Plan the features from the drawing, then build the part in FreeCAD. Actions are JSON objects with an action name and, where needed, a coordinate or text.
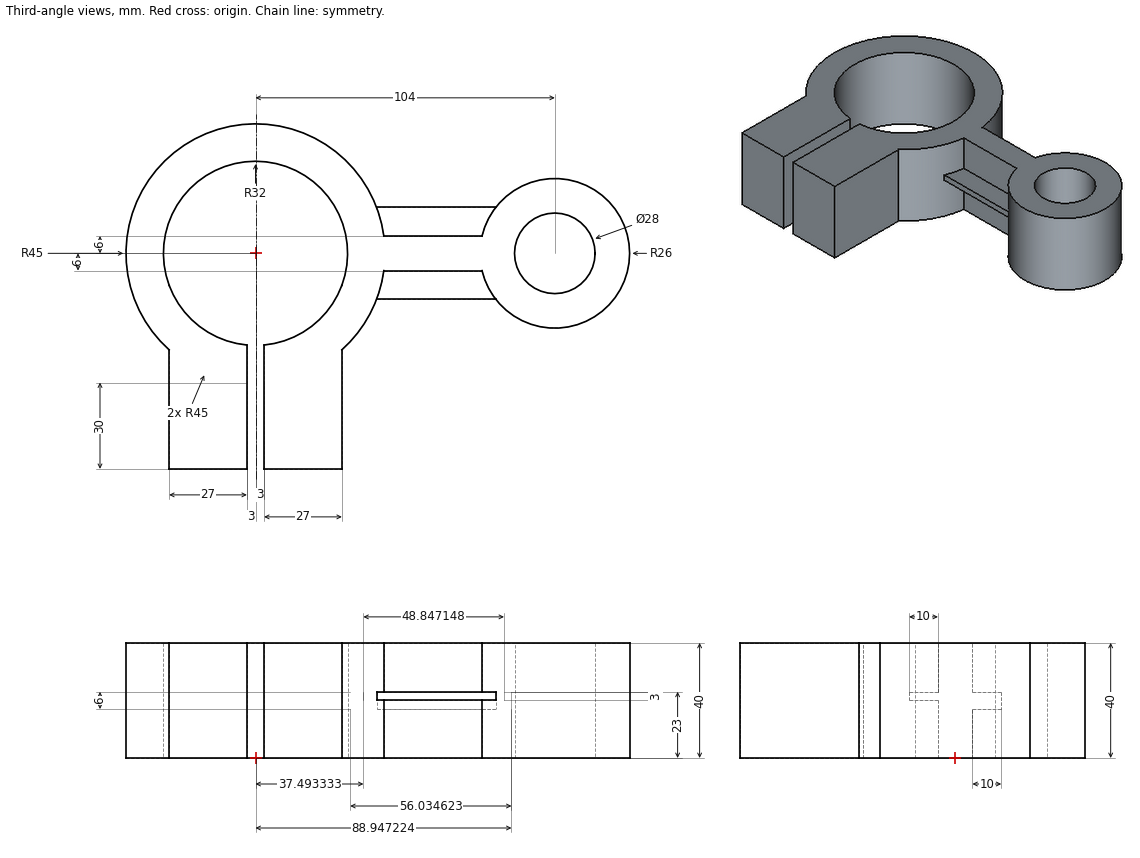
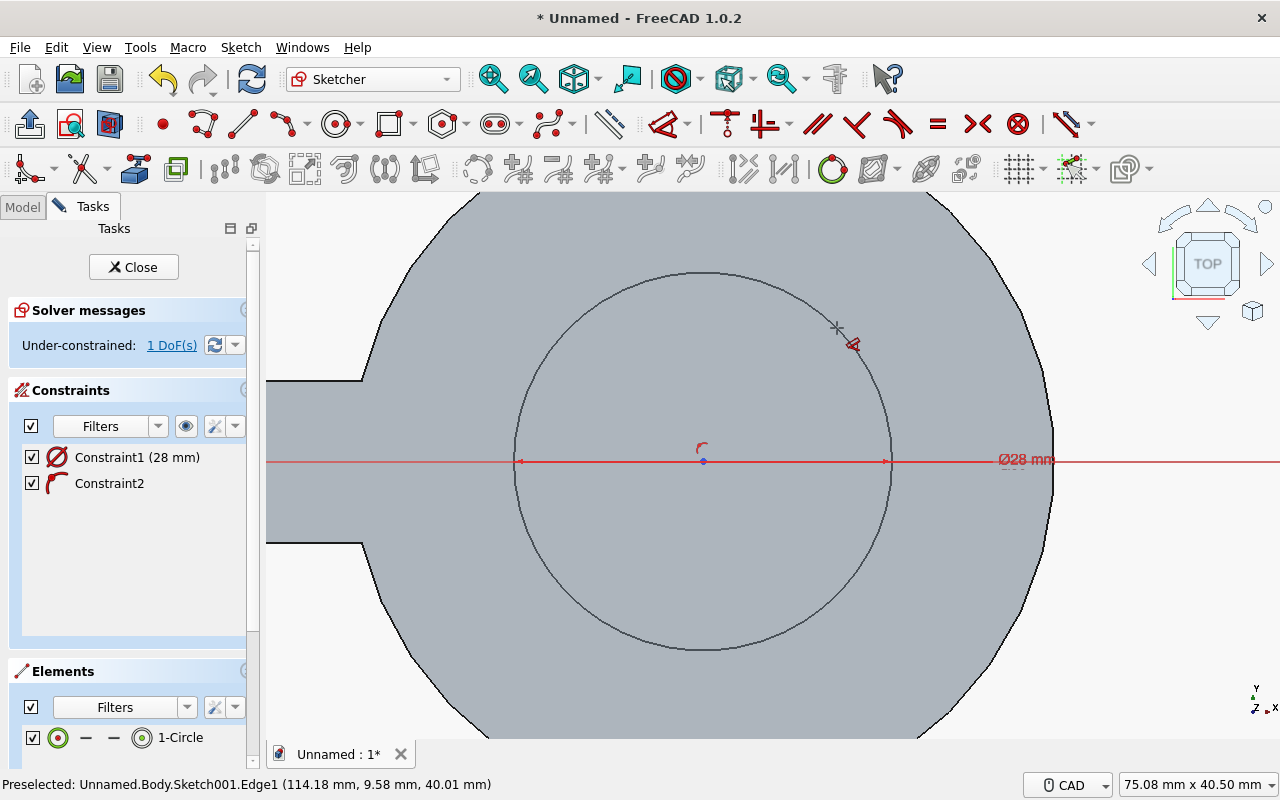
{"action": "left_click", "coordinate": [703, 462]}
{"action": "left_click", "coordinate": [498, 496]}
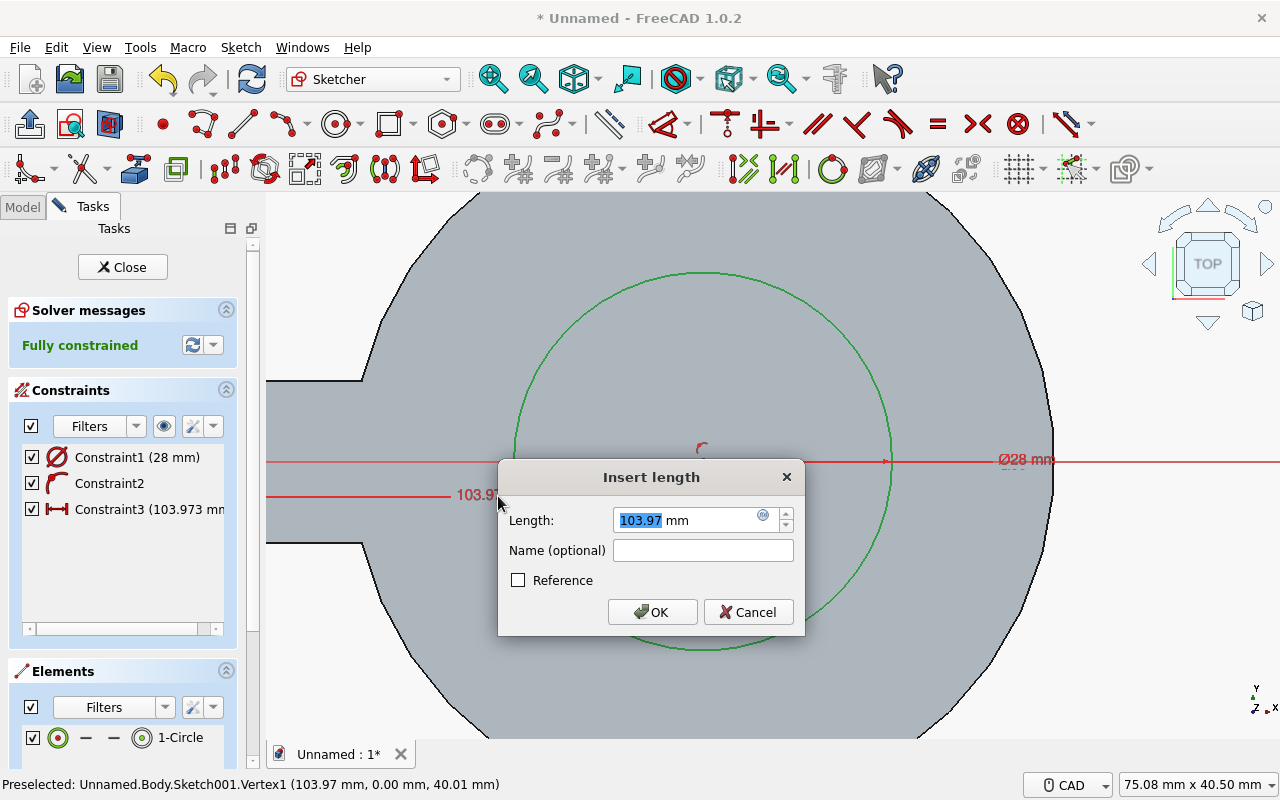
{"action": "type", "text": "104"}
{"action": "key", "text": "Return"}
{"action": "key", "text": "Escape"}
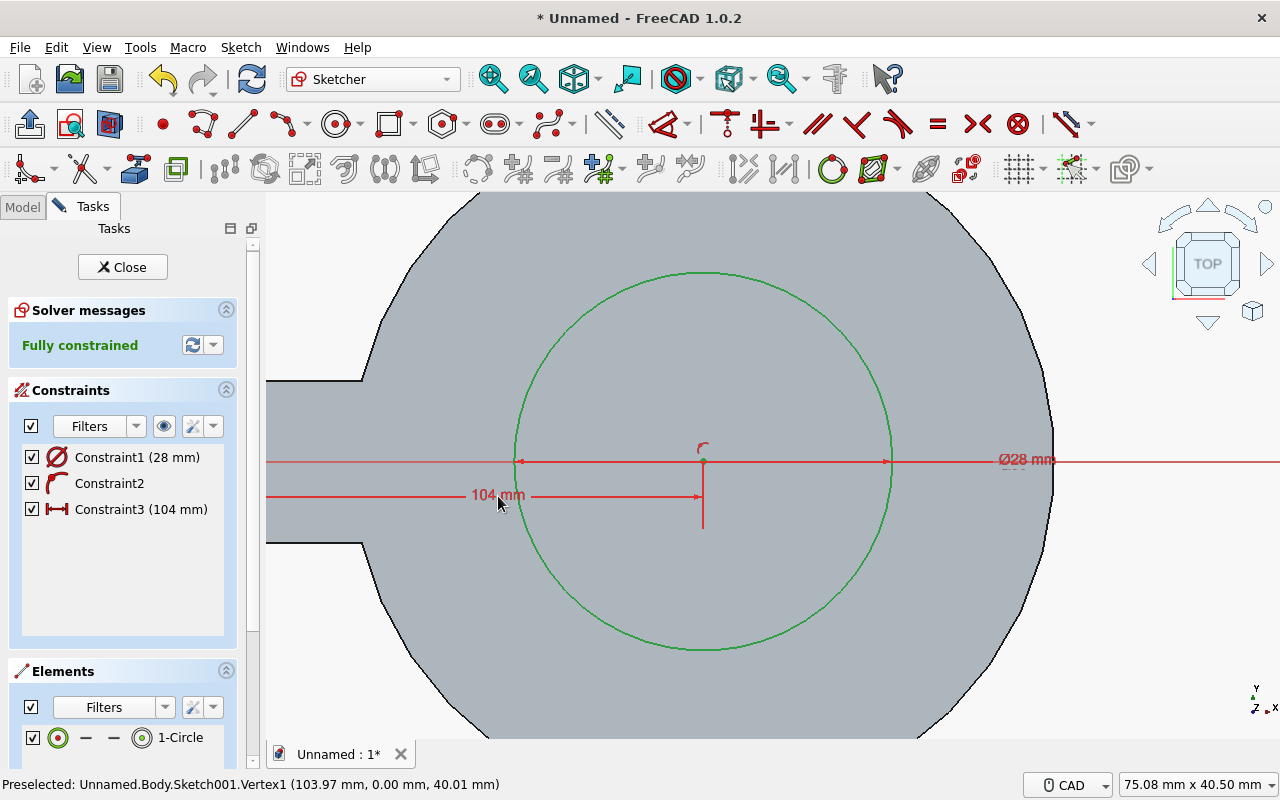
{"action": "left_click", "coordinate": [123, 267]}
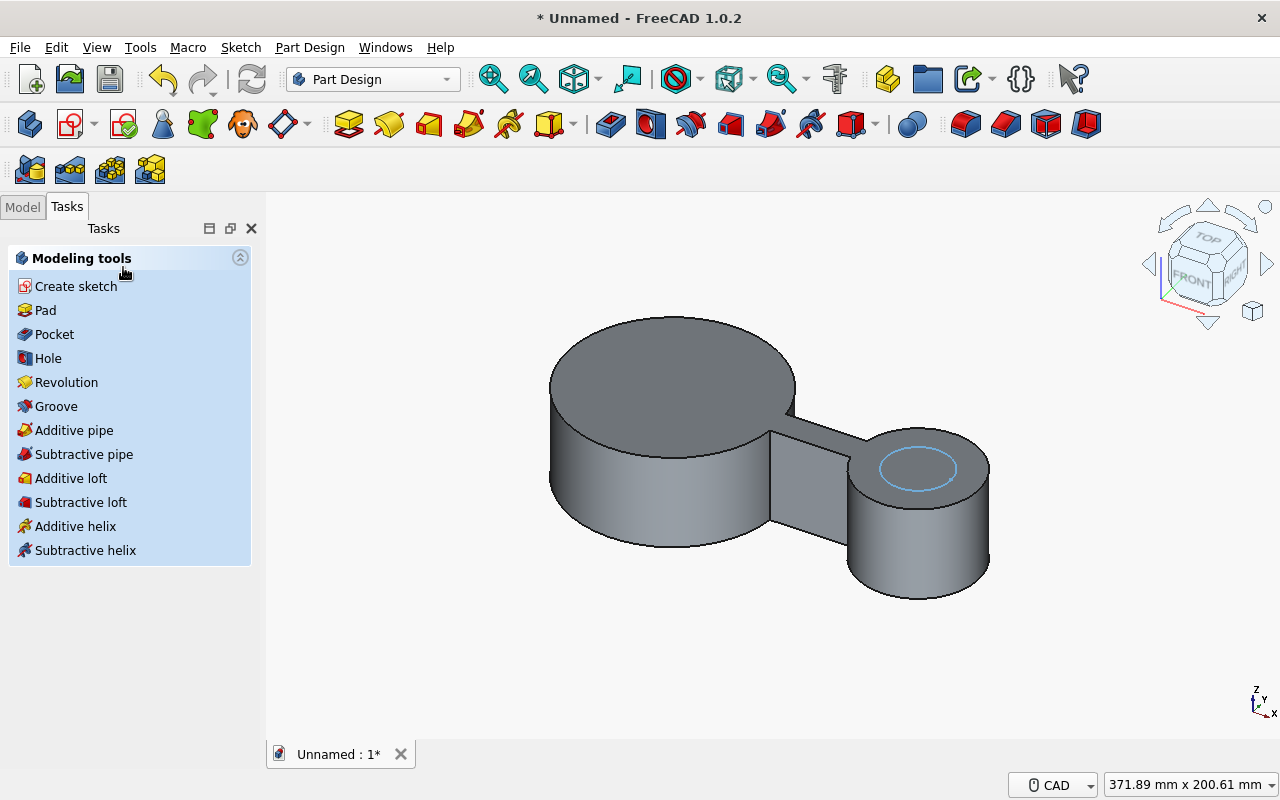
{"action": "left_click", "coordinate": [612, 124]}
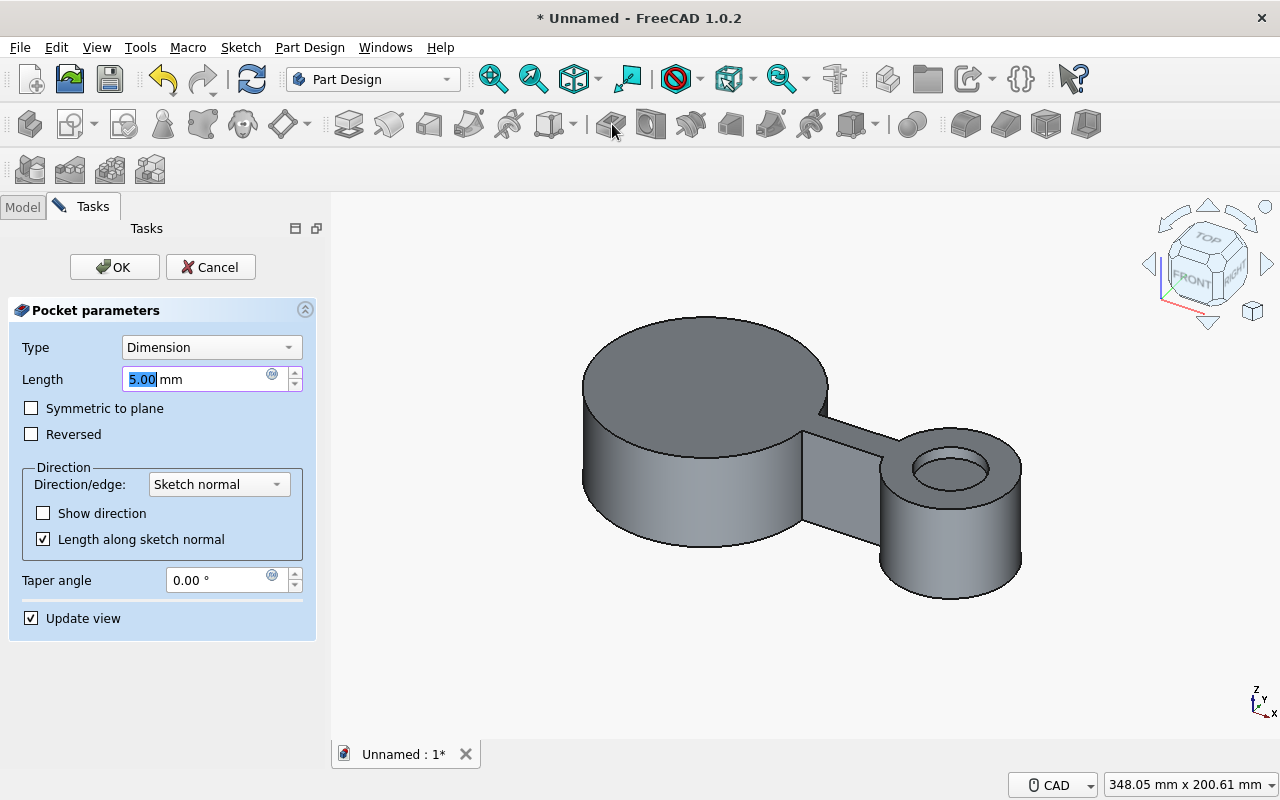
{"action": "type", "text": "40"}
{"action": "key", "text": "Tab"}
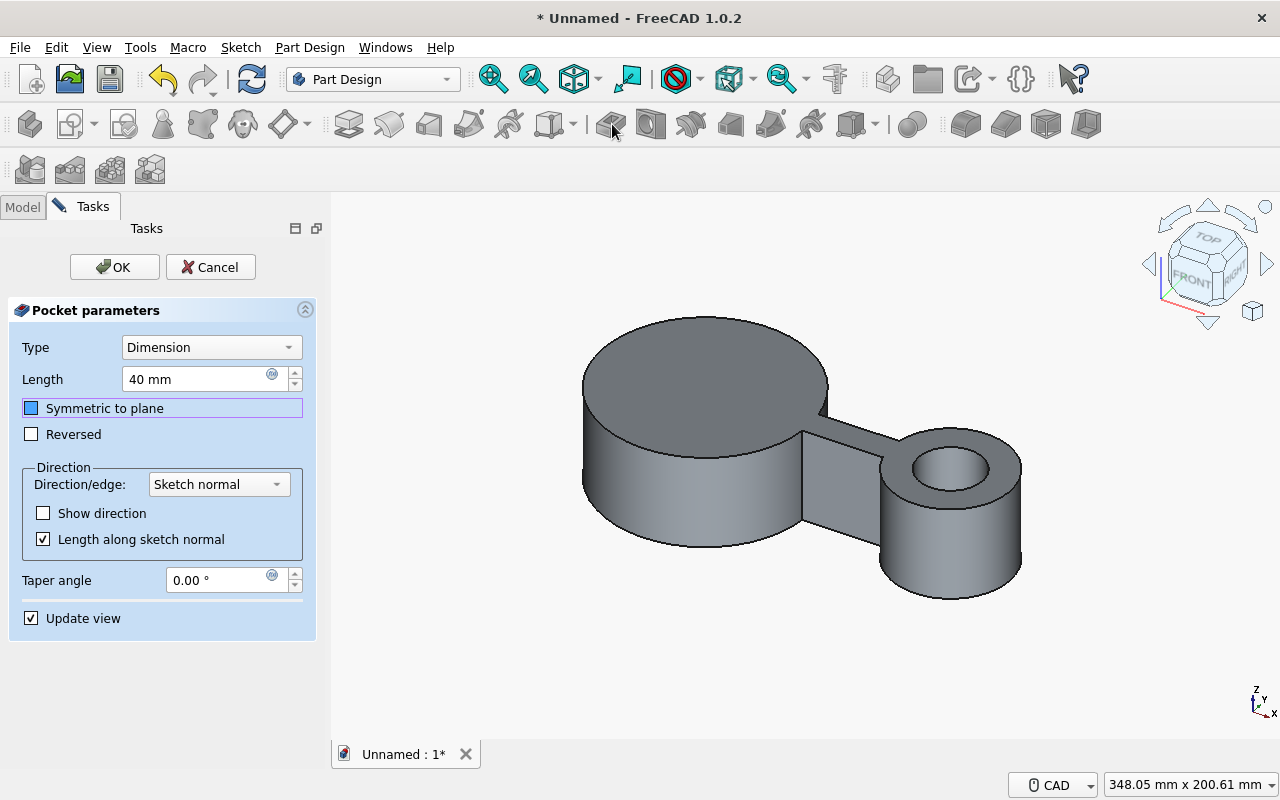
{"action": "left_click", "coordinate": [115, 267]}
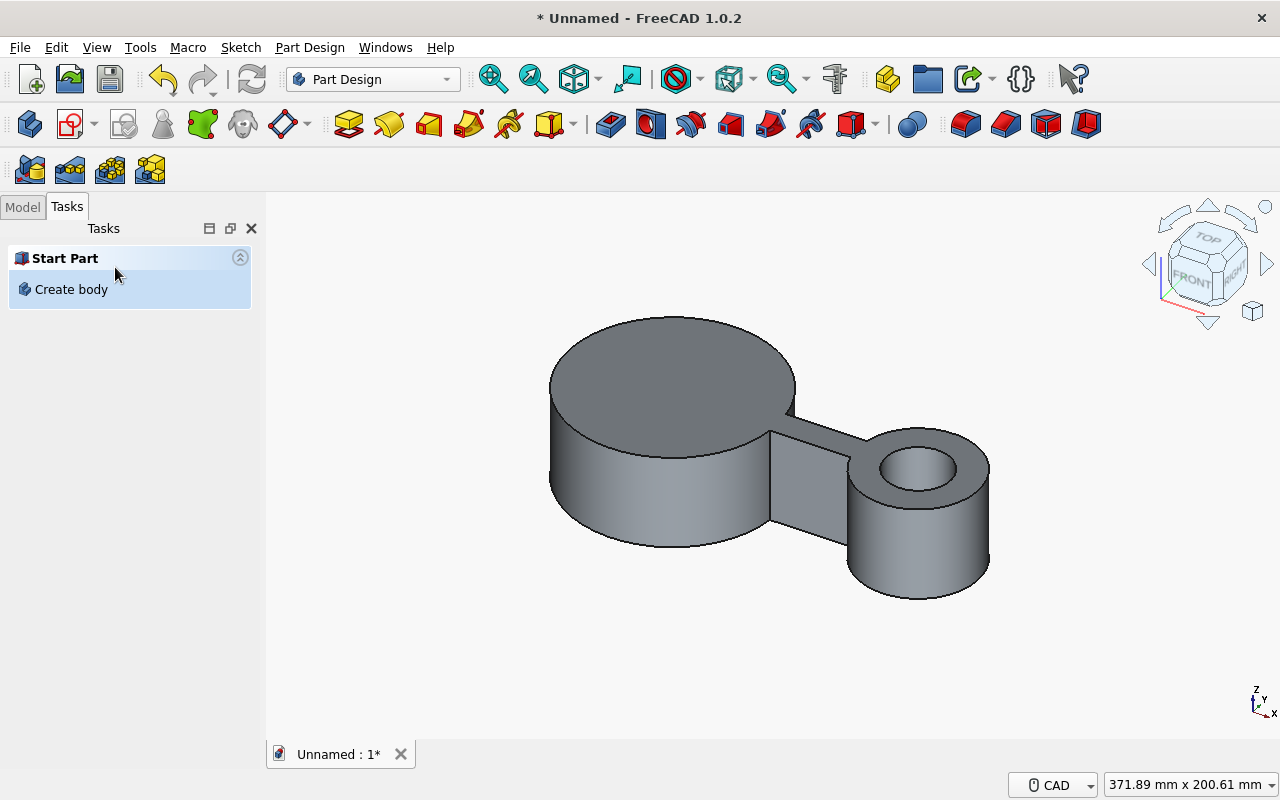
{"action": "key", "text": "5"}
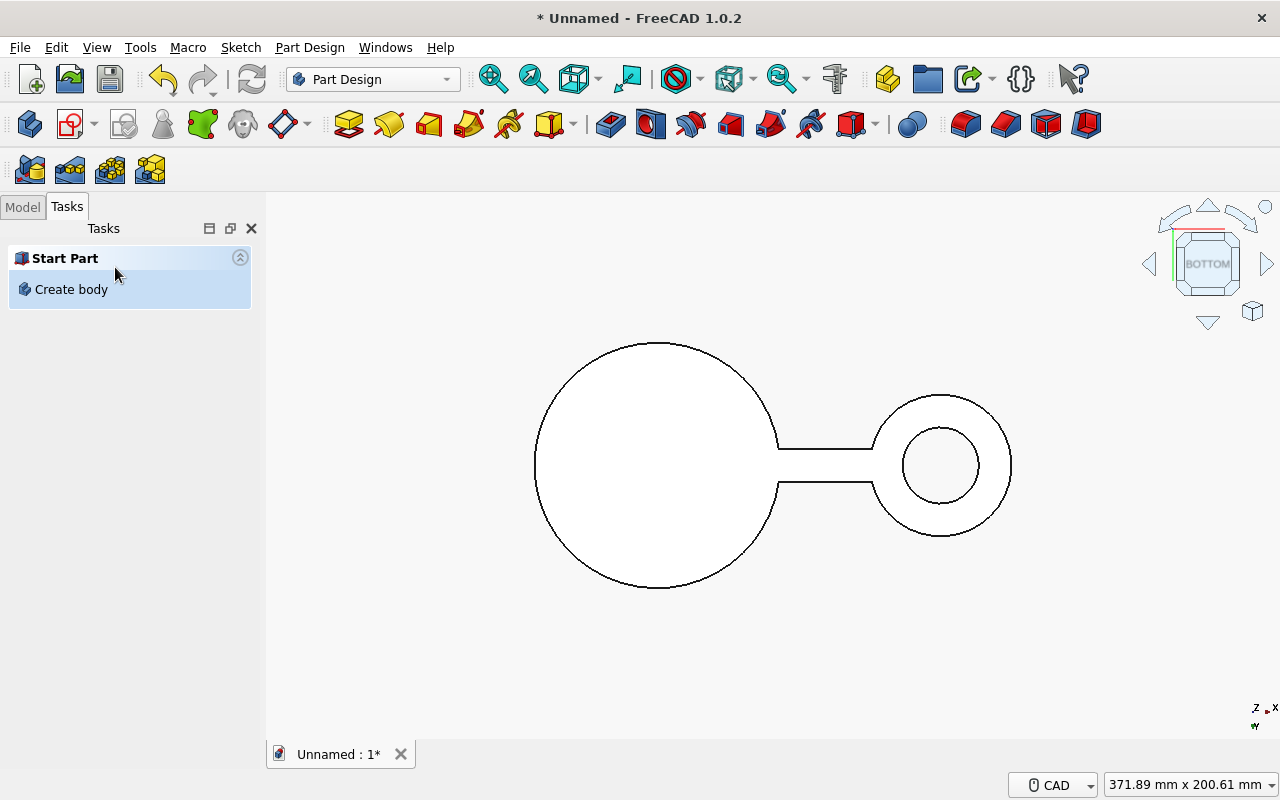
{"action": "left_click", "coordinate": [637, 464]}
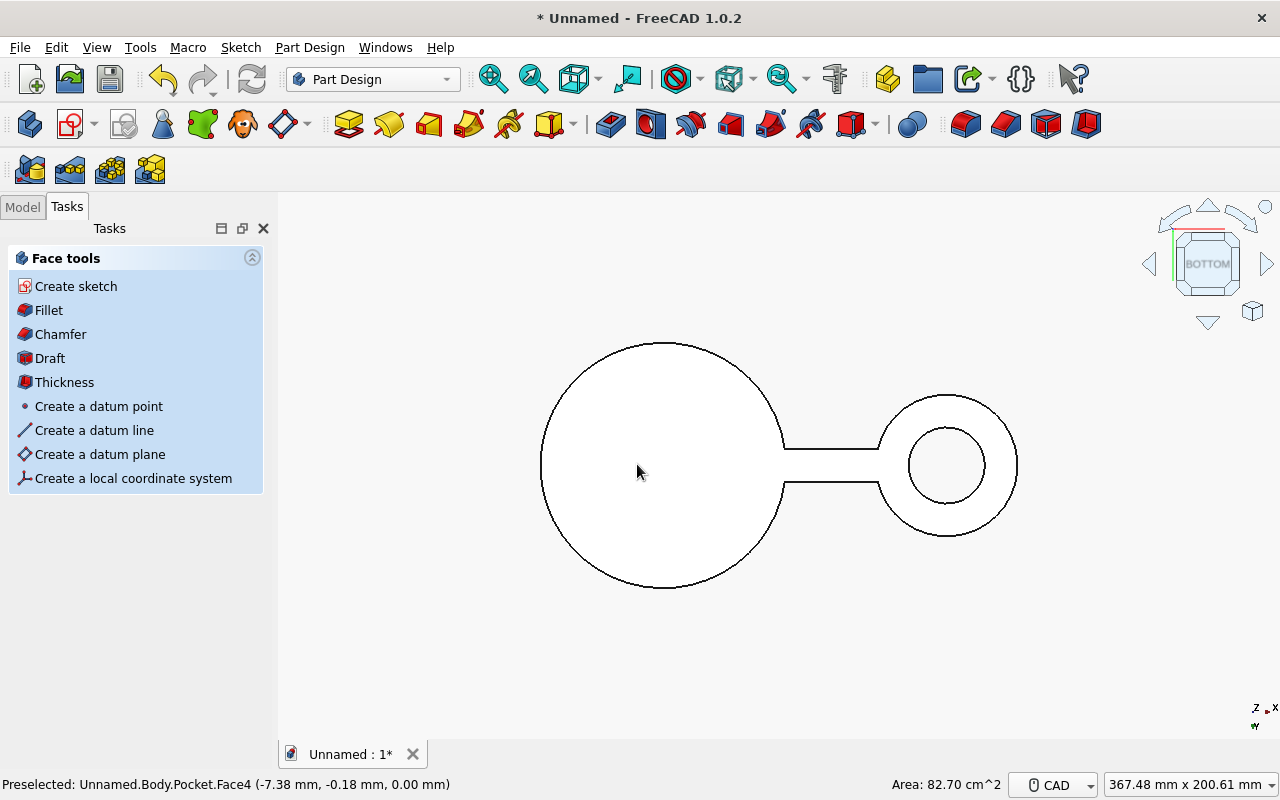
{"action": "left_click", "coordinate": [70, 124]}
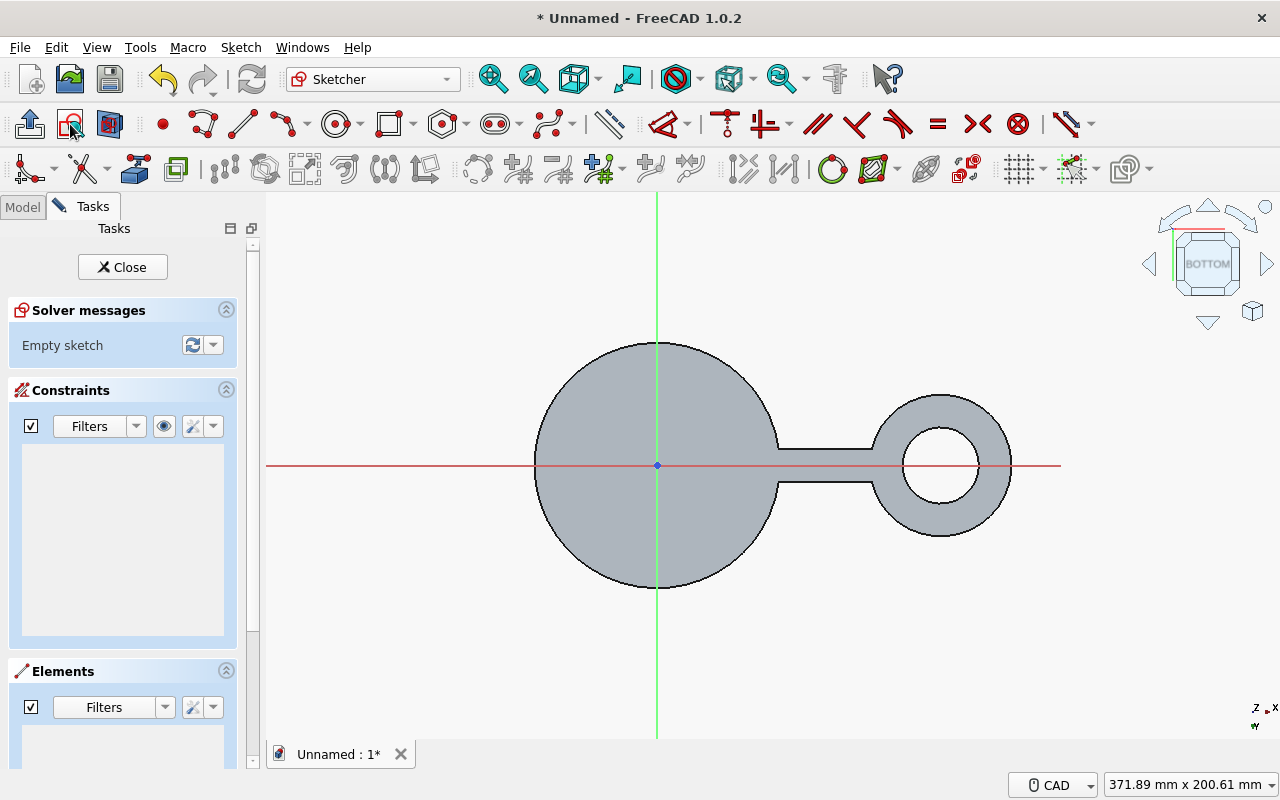
{"action": "scroll", "coordinate": [599, 426], "scroll_direction": "up", "scroll_amount": 3}